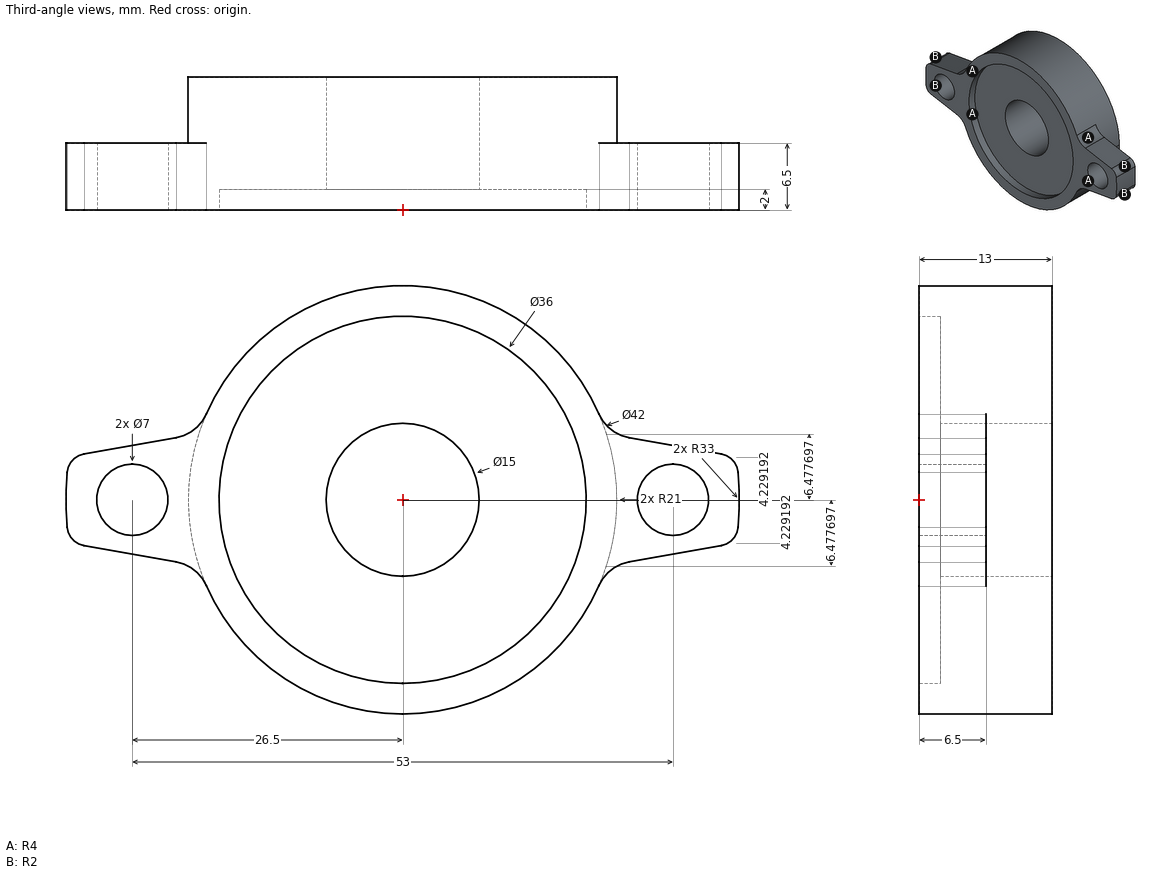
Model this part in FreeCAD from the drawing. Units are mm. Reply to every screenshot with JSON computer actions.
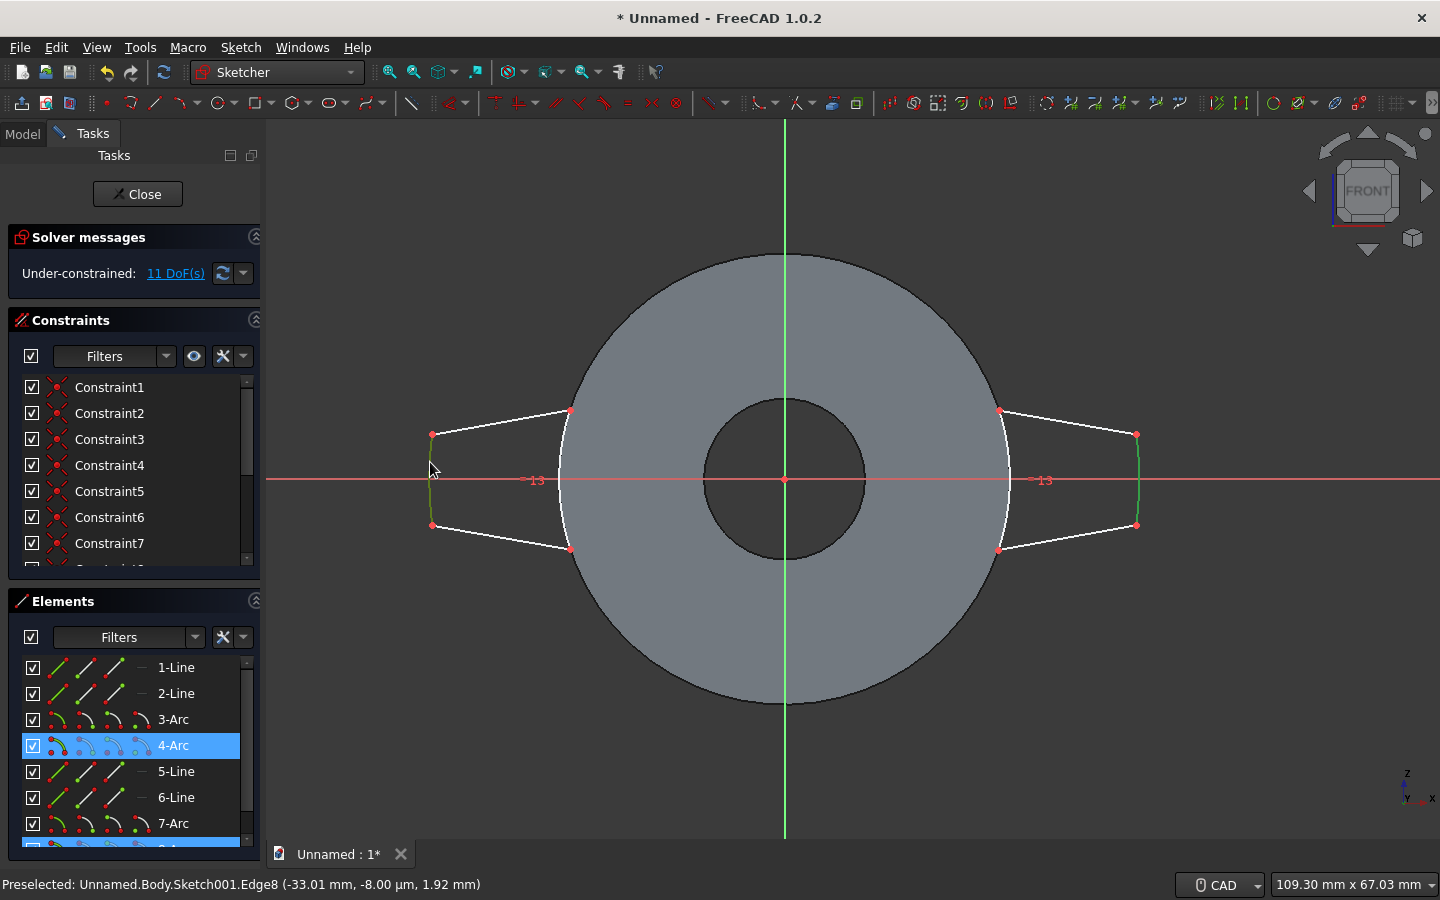
{"action": "left_click", "coordinate": [628, 104]}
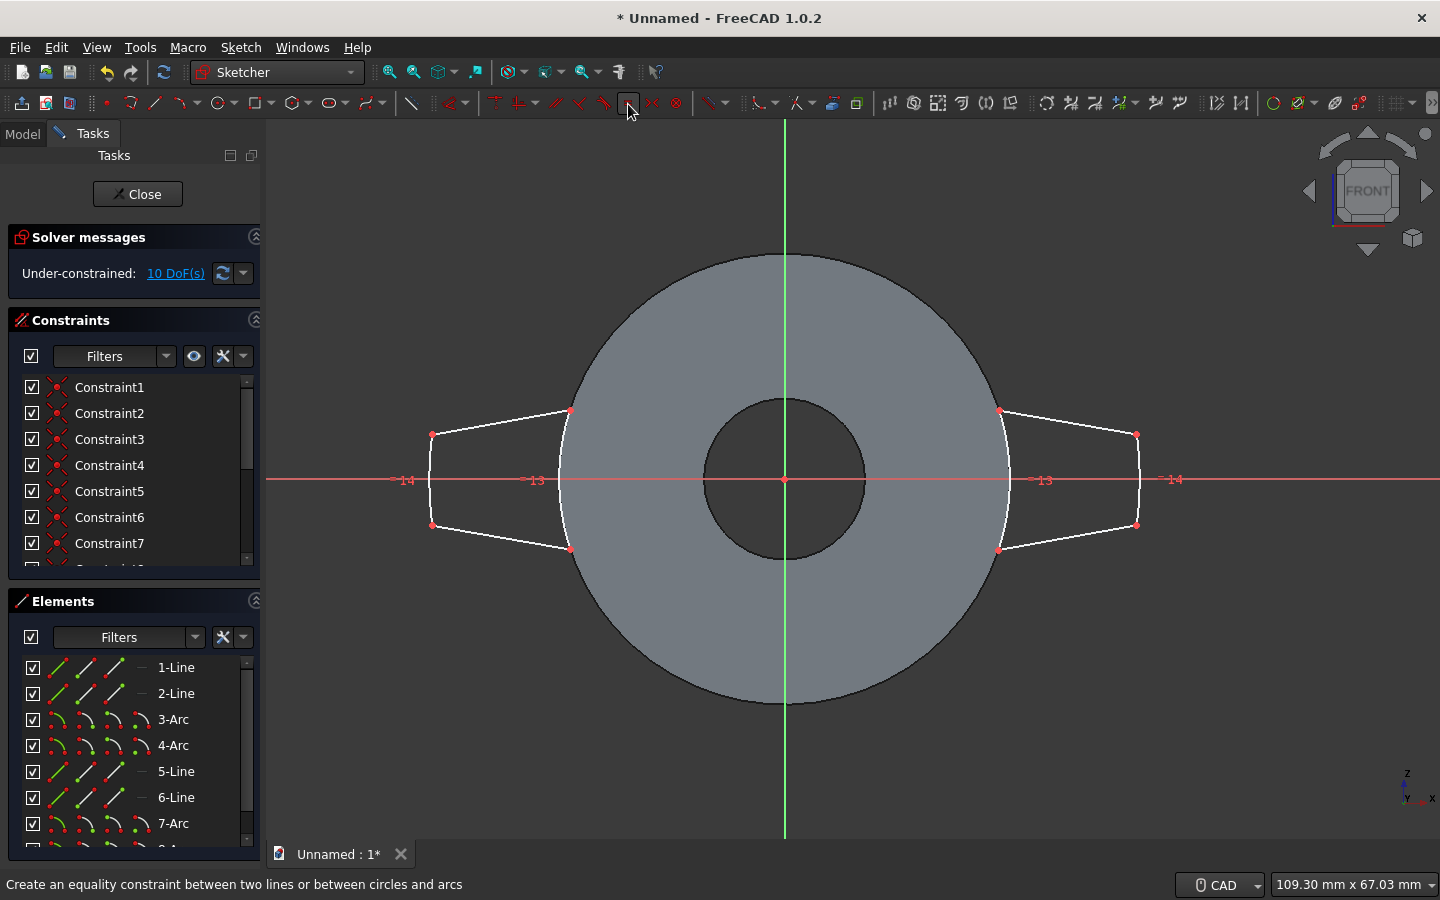
{"action": "left_click", "coordinate": [450, 104]}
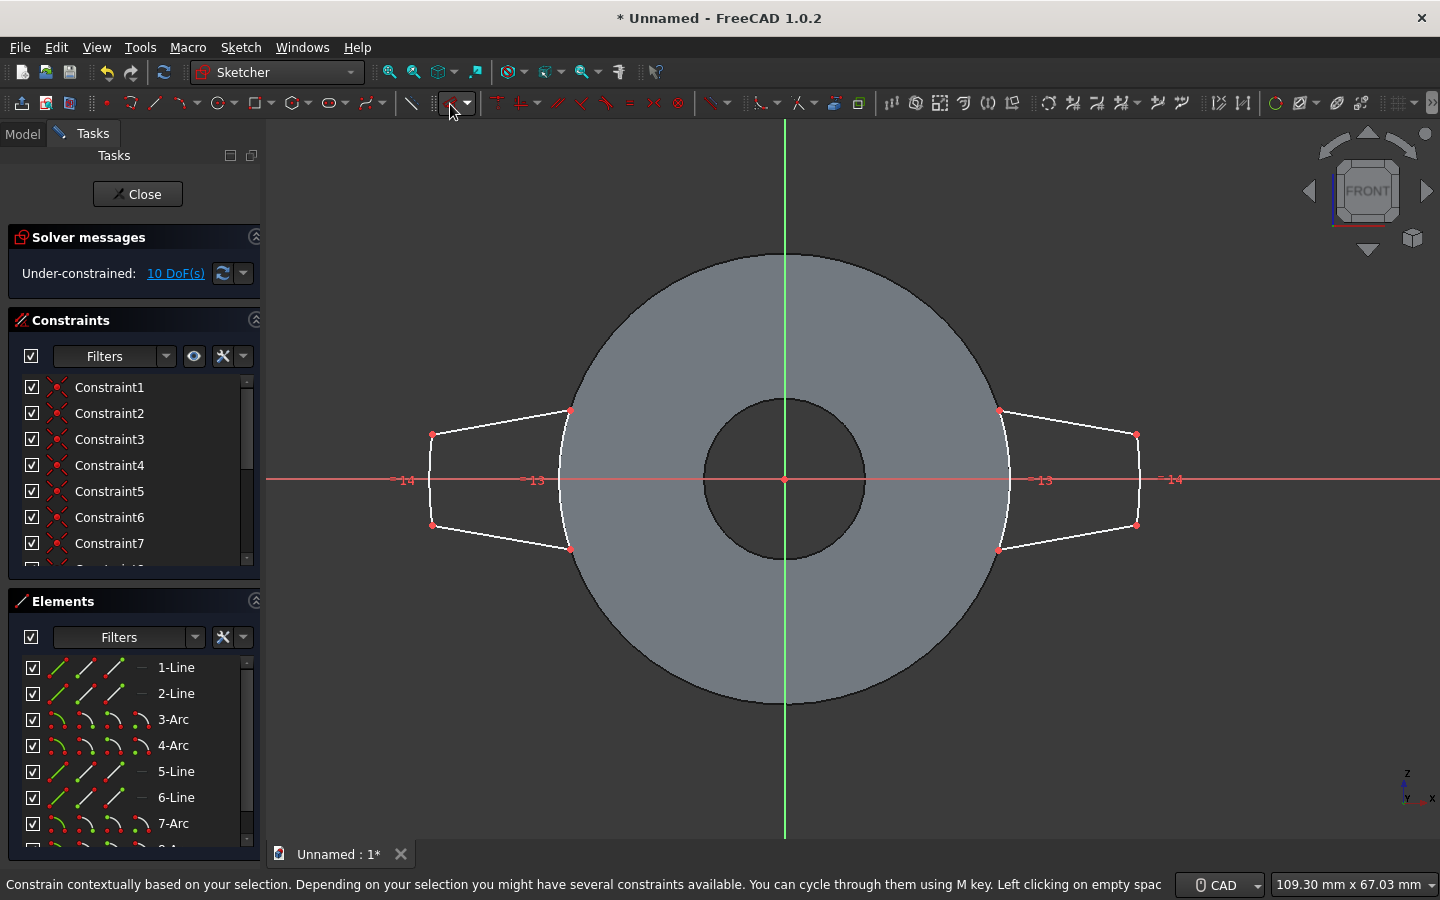
{"action": "left_click", "coordinate": [1008, 509]}
{"action": "left_click", "coordinate": [1040, 513]}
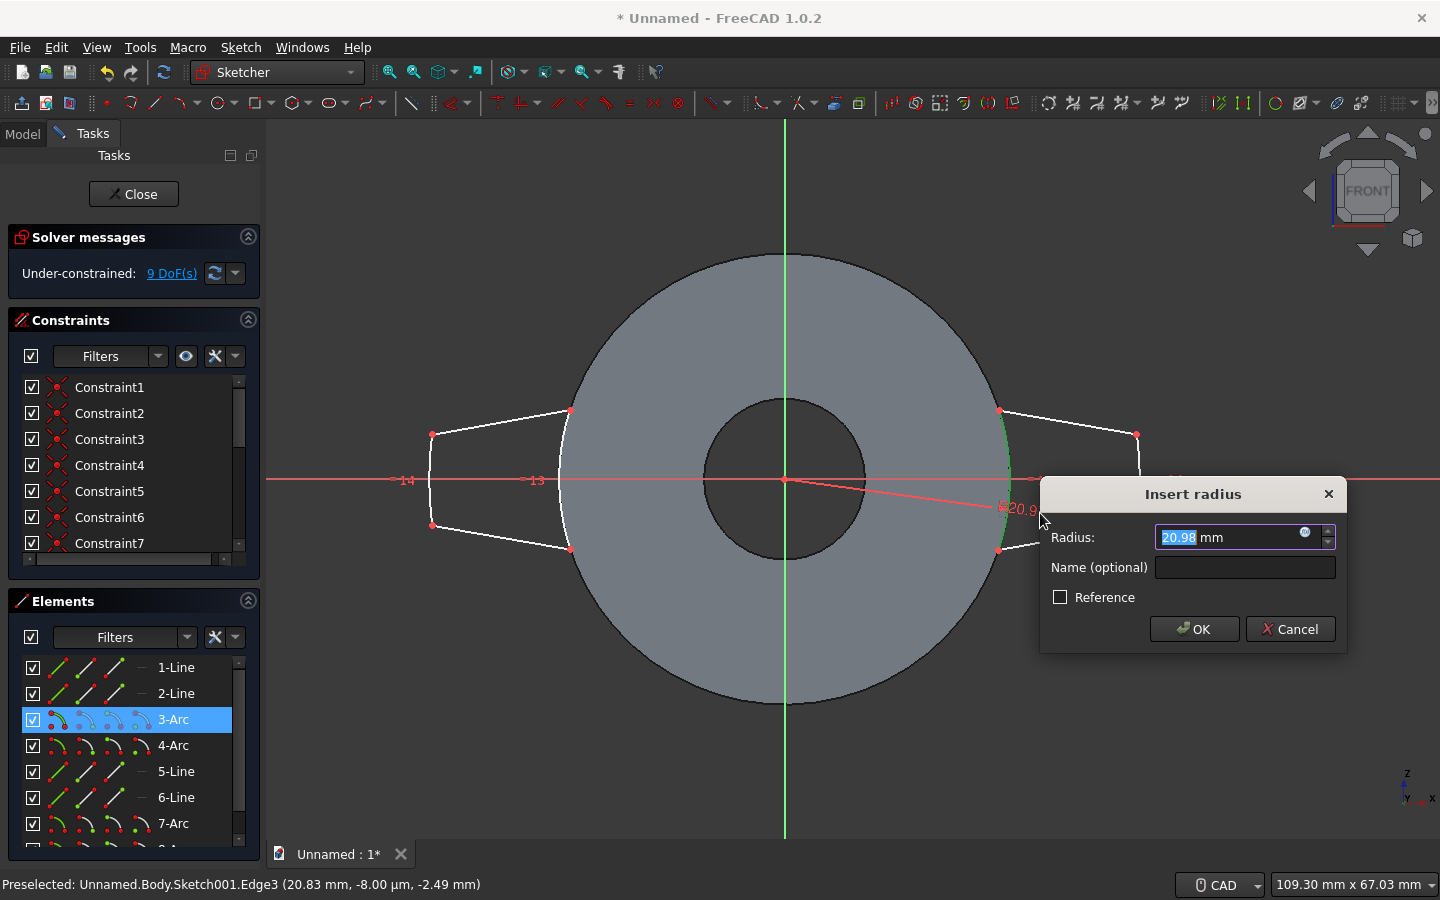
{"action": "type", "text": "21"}
{"action": "key", "text": "Return"}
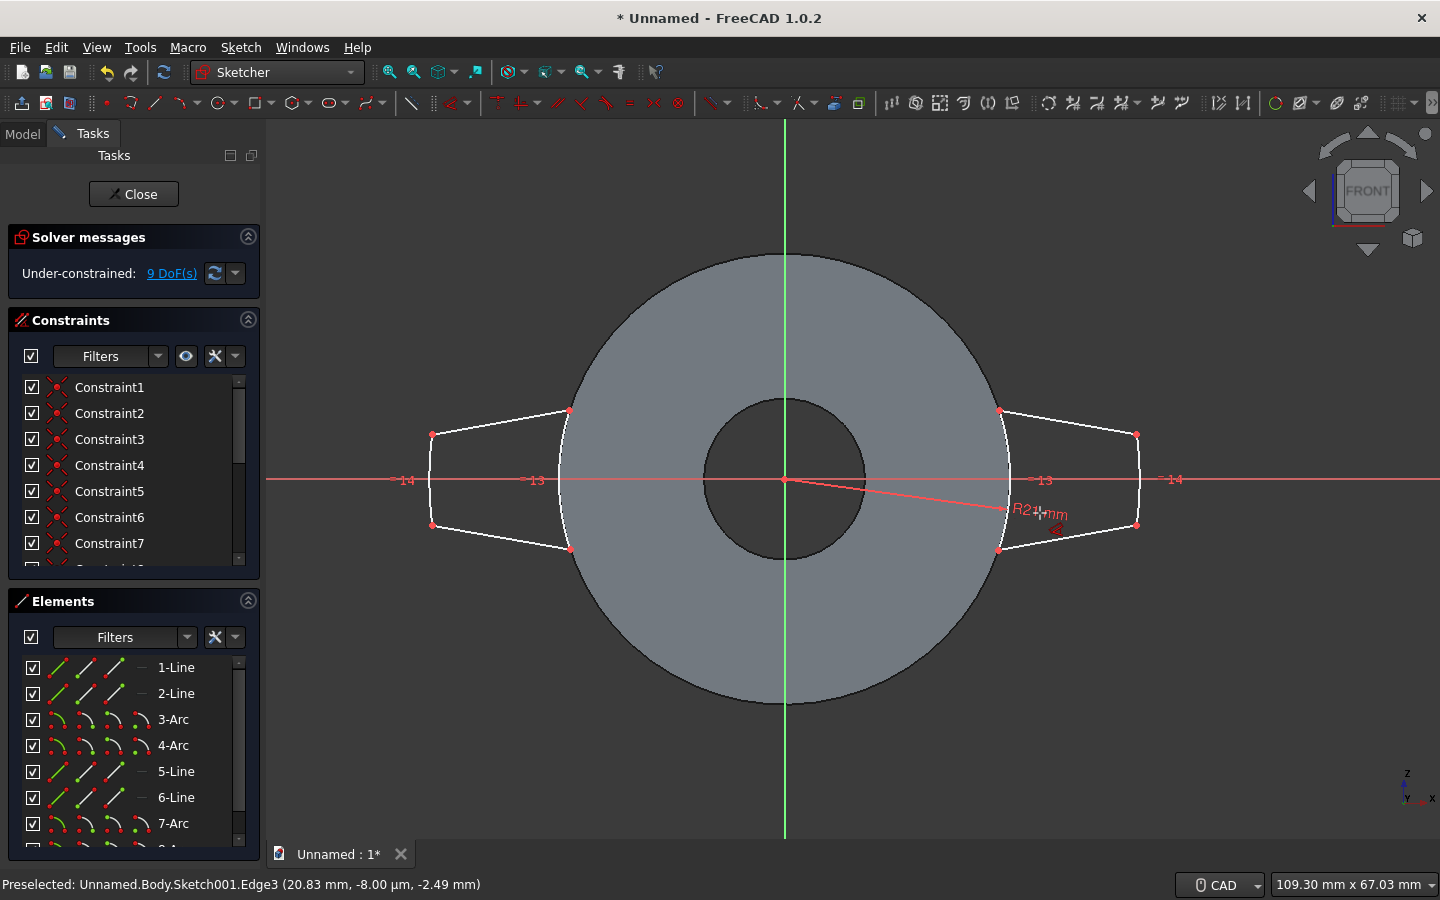
{"action": "left_click", "coordinate": [1139, 498]}
{"action": "left_click", "coordinate": [1171, 500]}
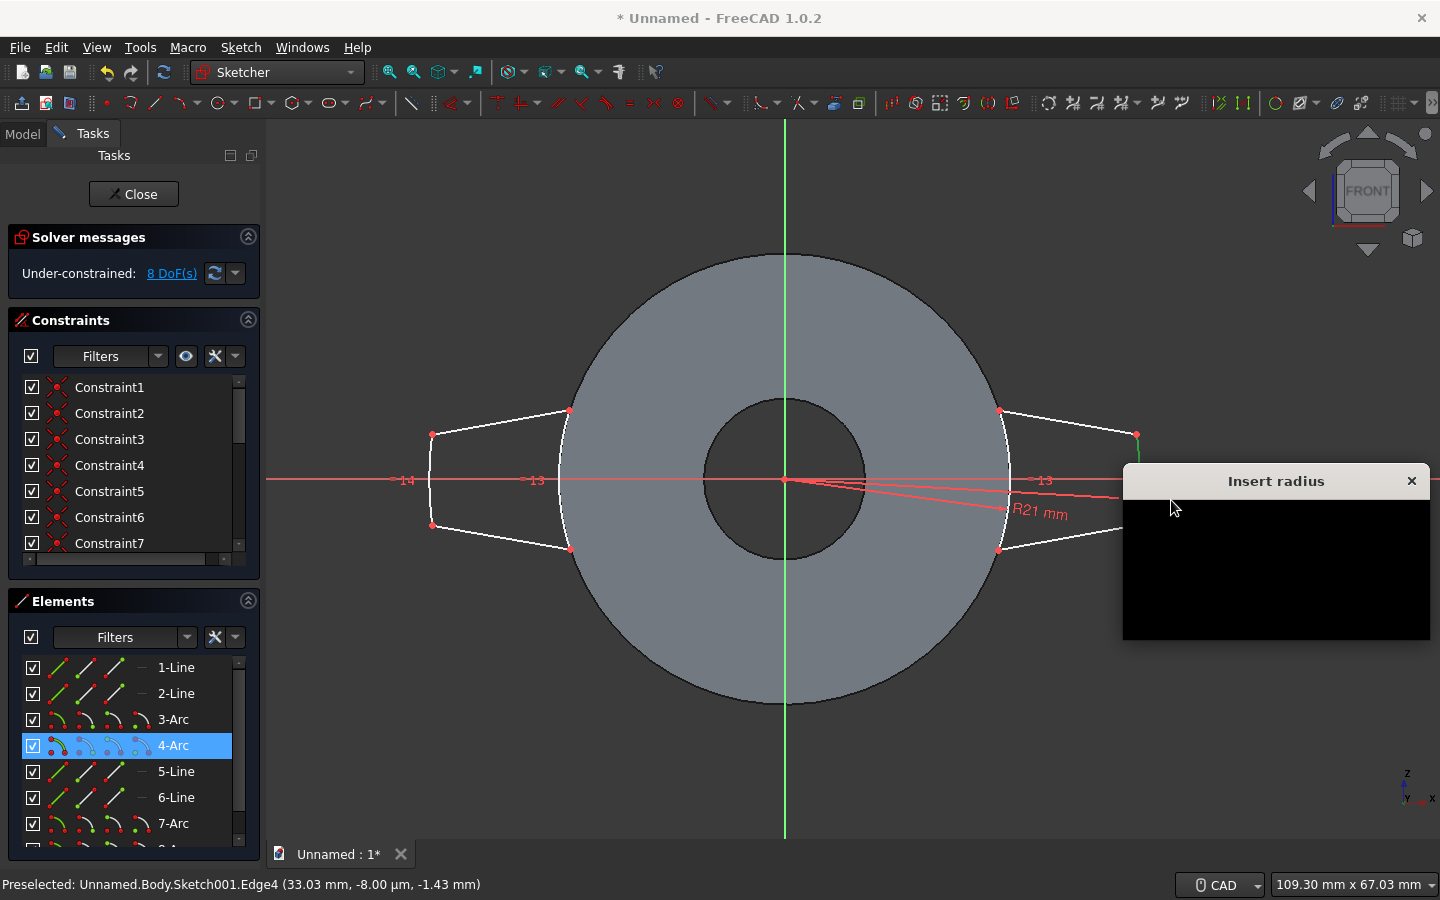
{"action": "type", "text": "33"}
{"action": "key", "text": "Return"}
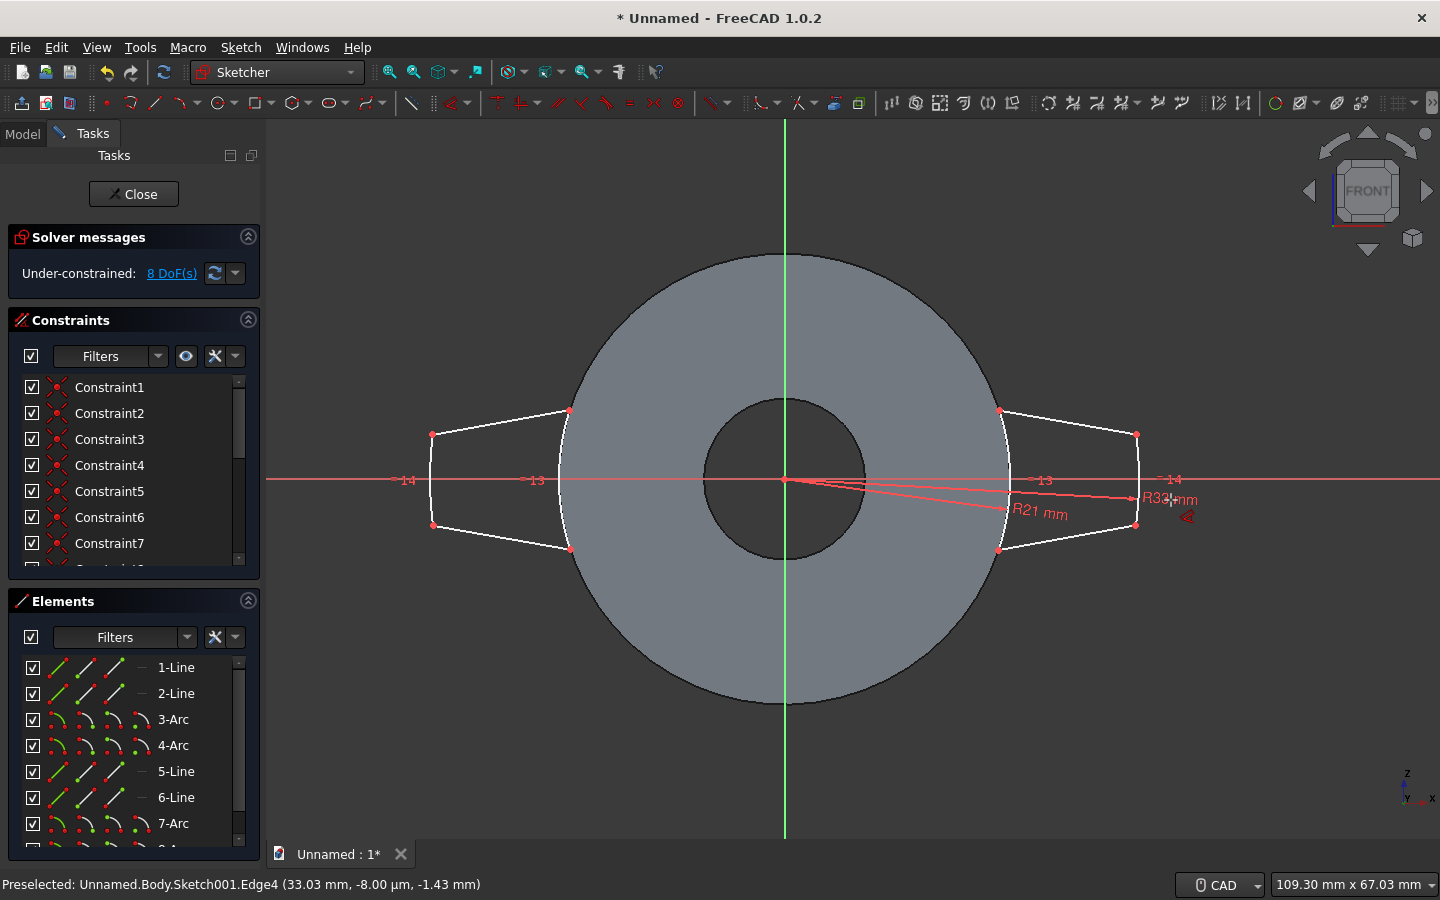
{"action": "left_click", "coordinate": [1136, 434]}
{"action": "left_click", "coordinate": [1170, 457]}